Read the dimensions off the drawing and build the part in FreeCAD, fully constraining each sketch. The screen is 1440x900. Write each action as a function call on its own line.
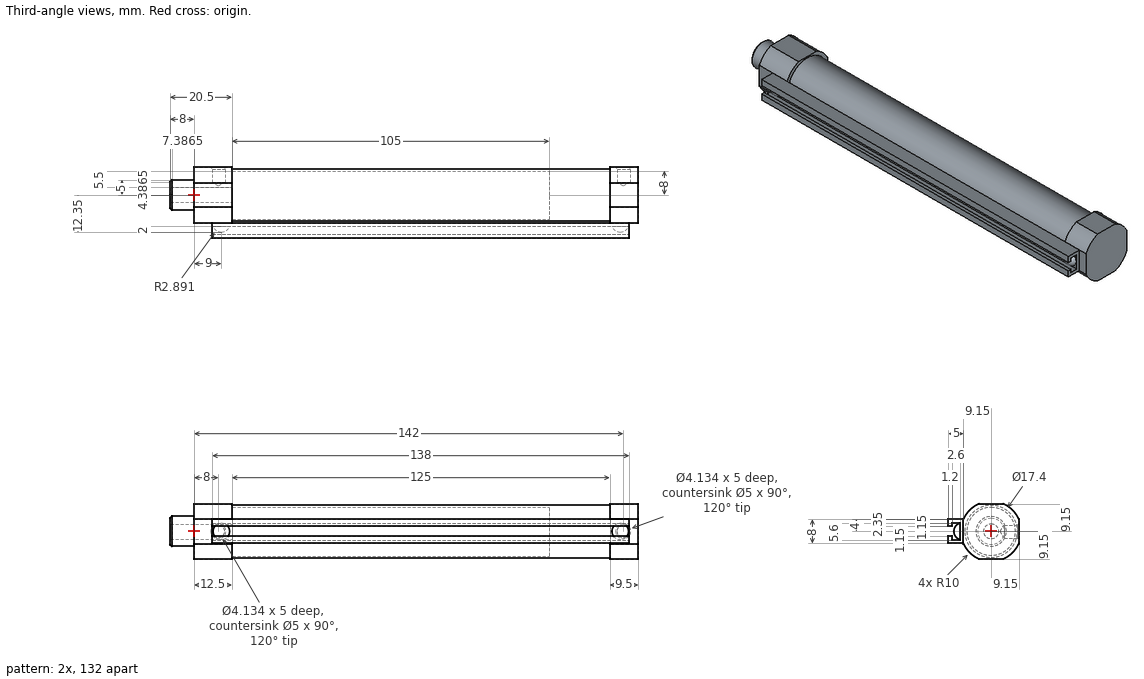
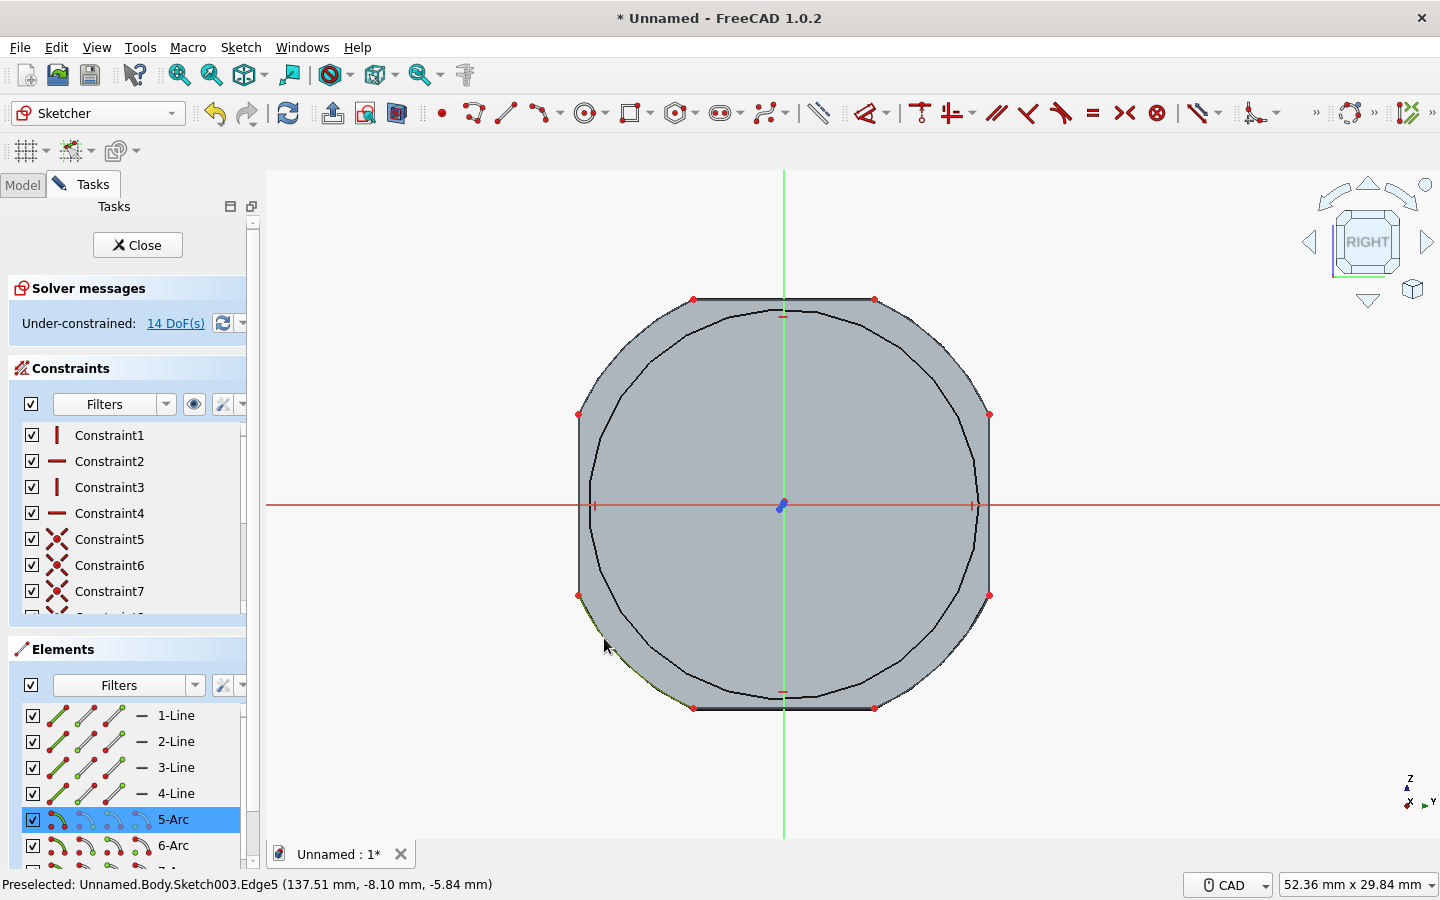
click(964, 372)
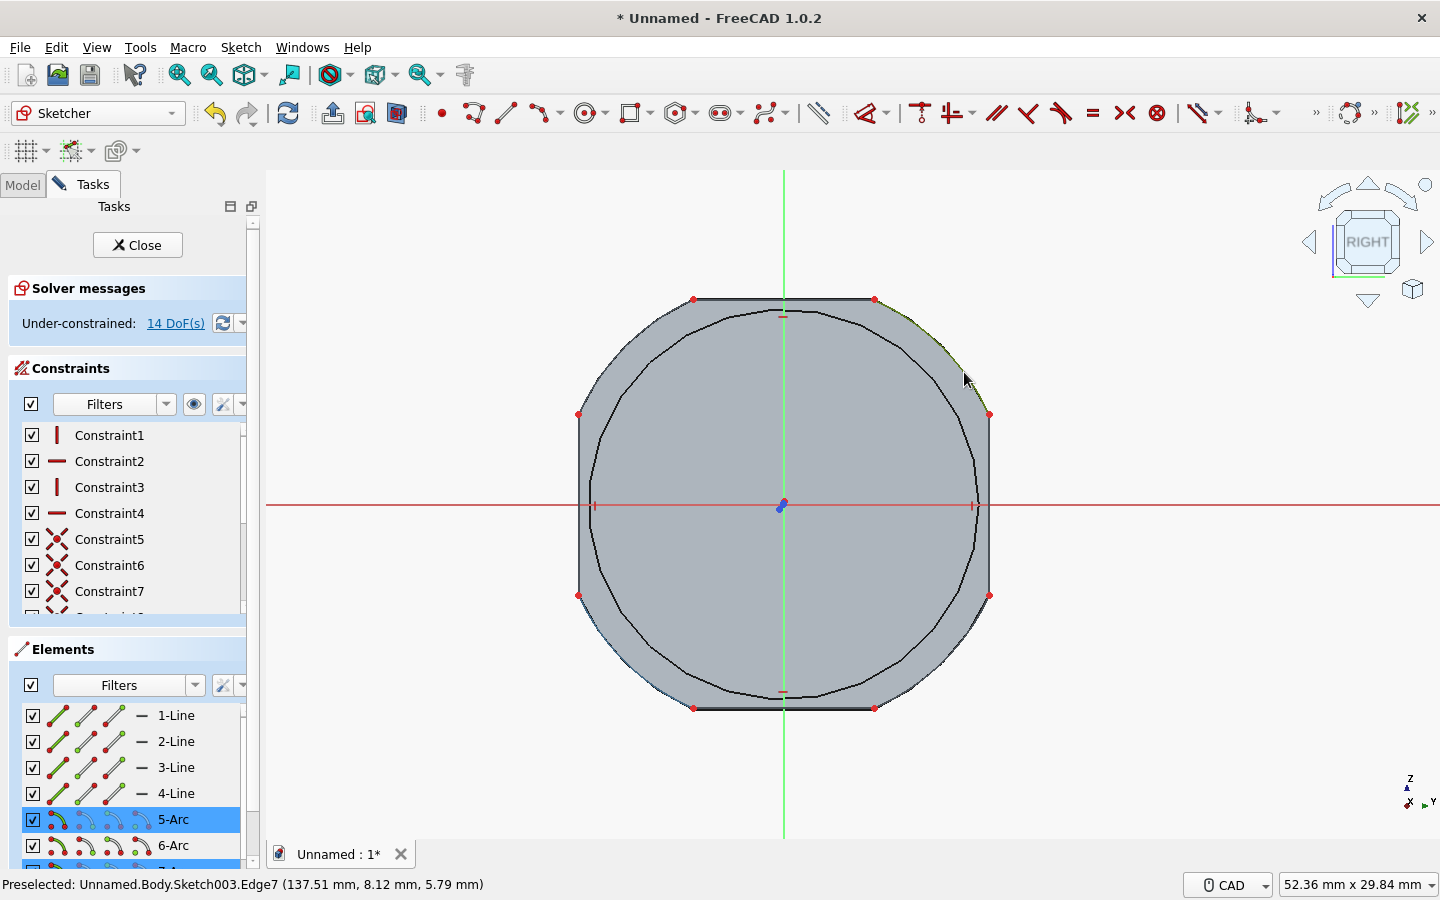
click(920, 114)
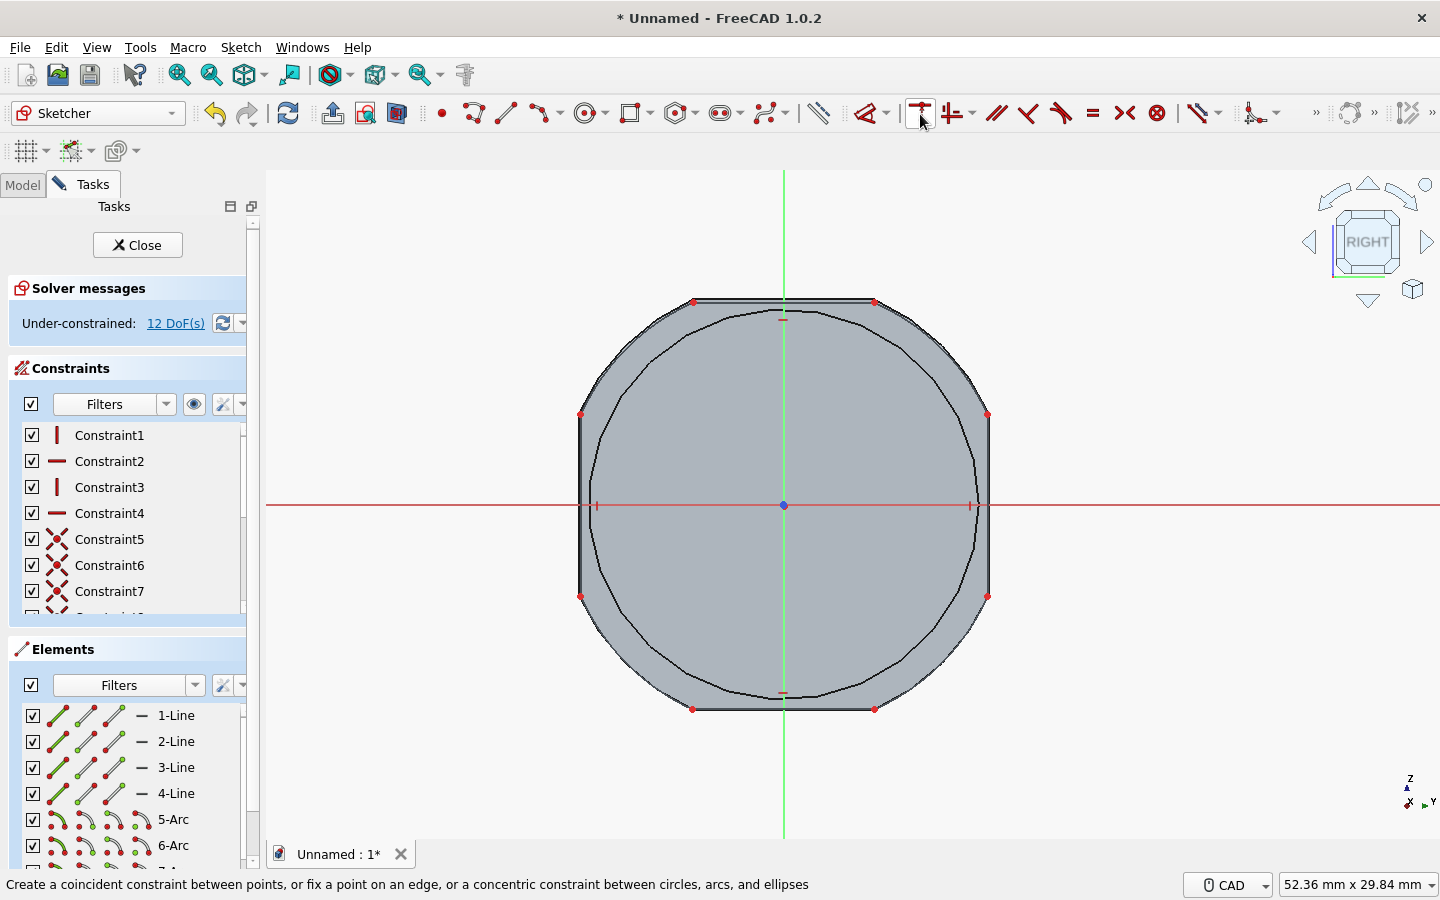
click(605, 638)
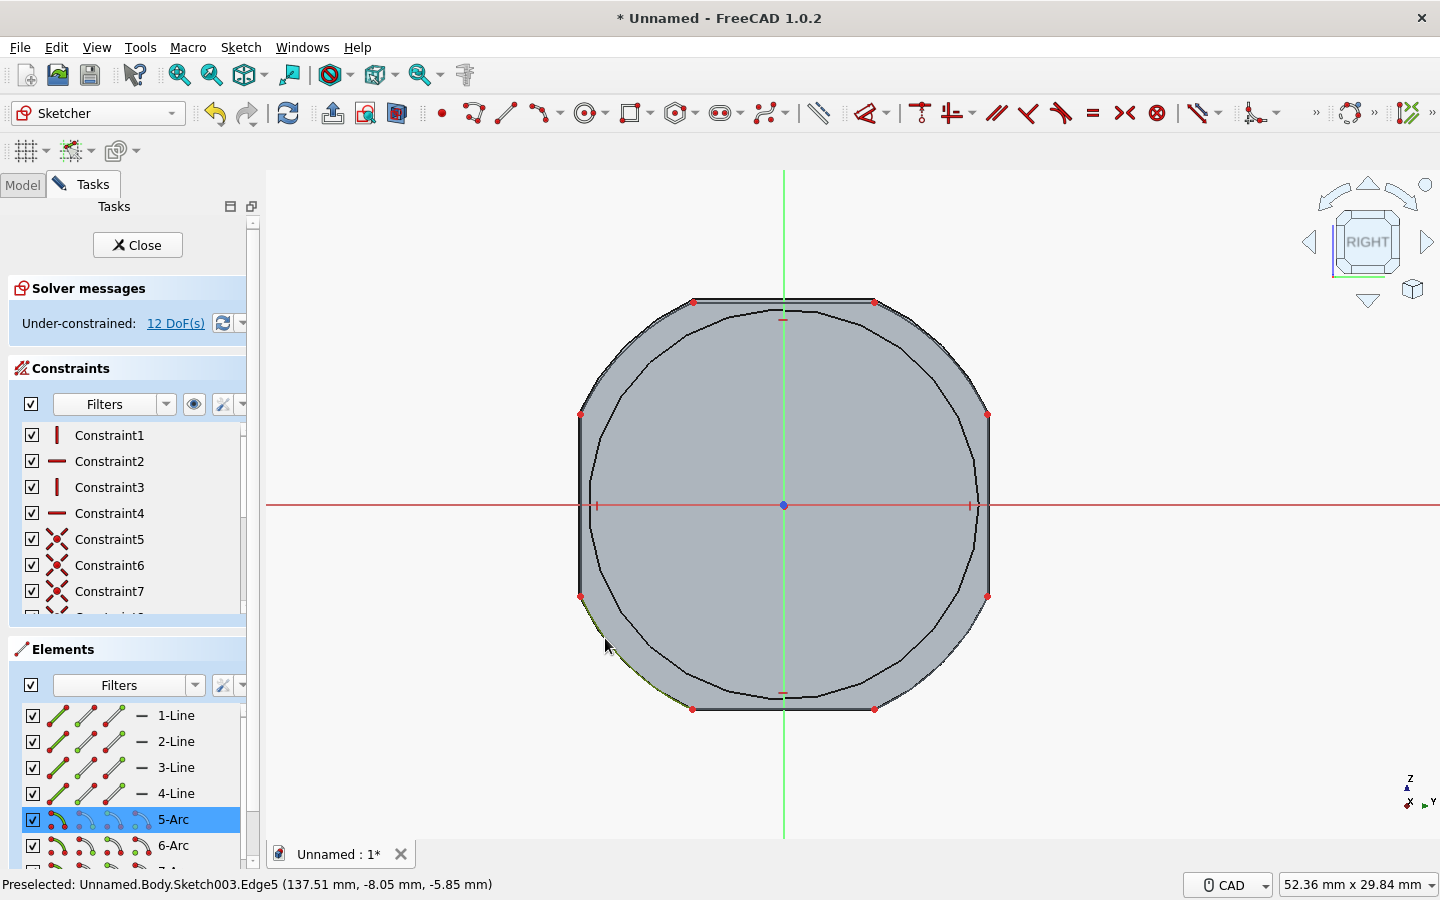
click(651, 327)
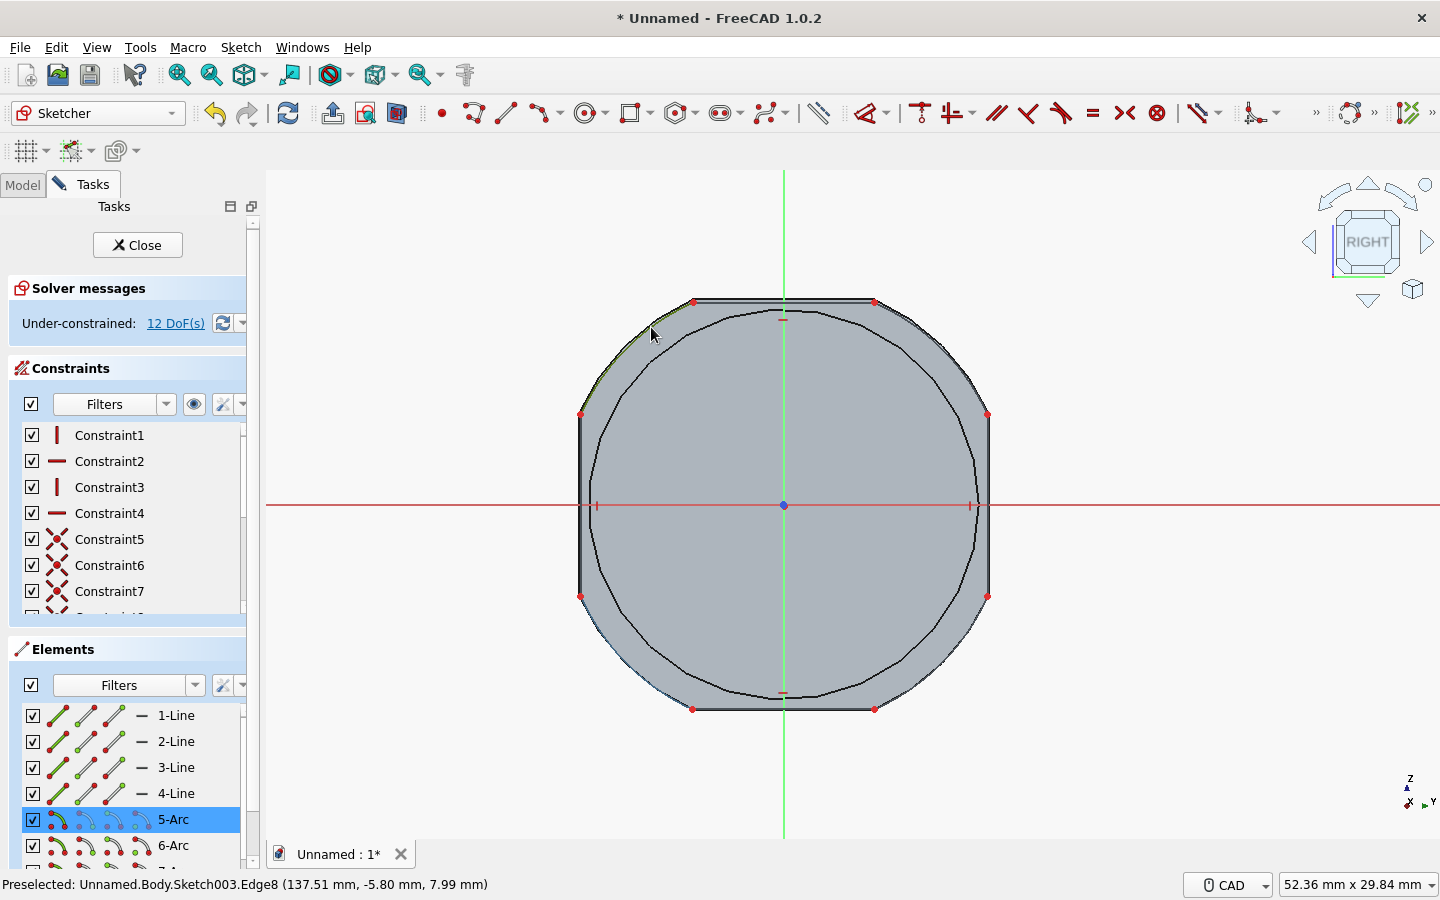
click(920, 114)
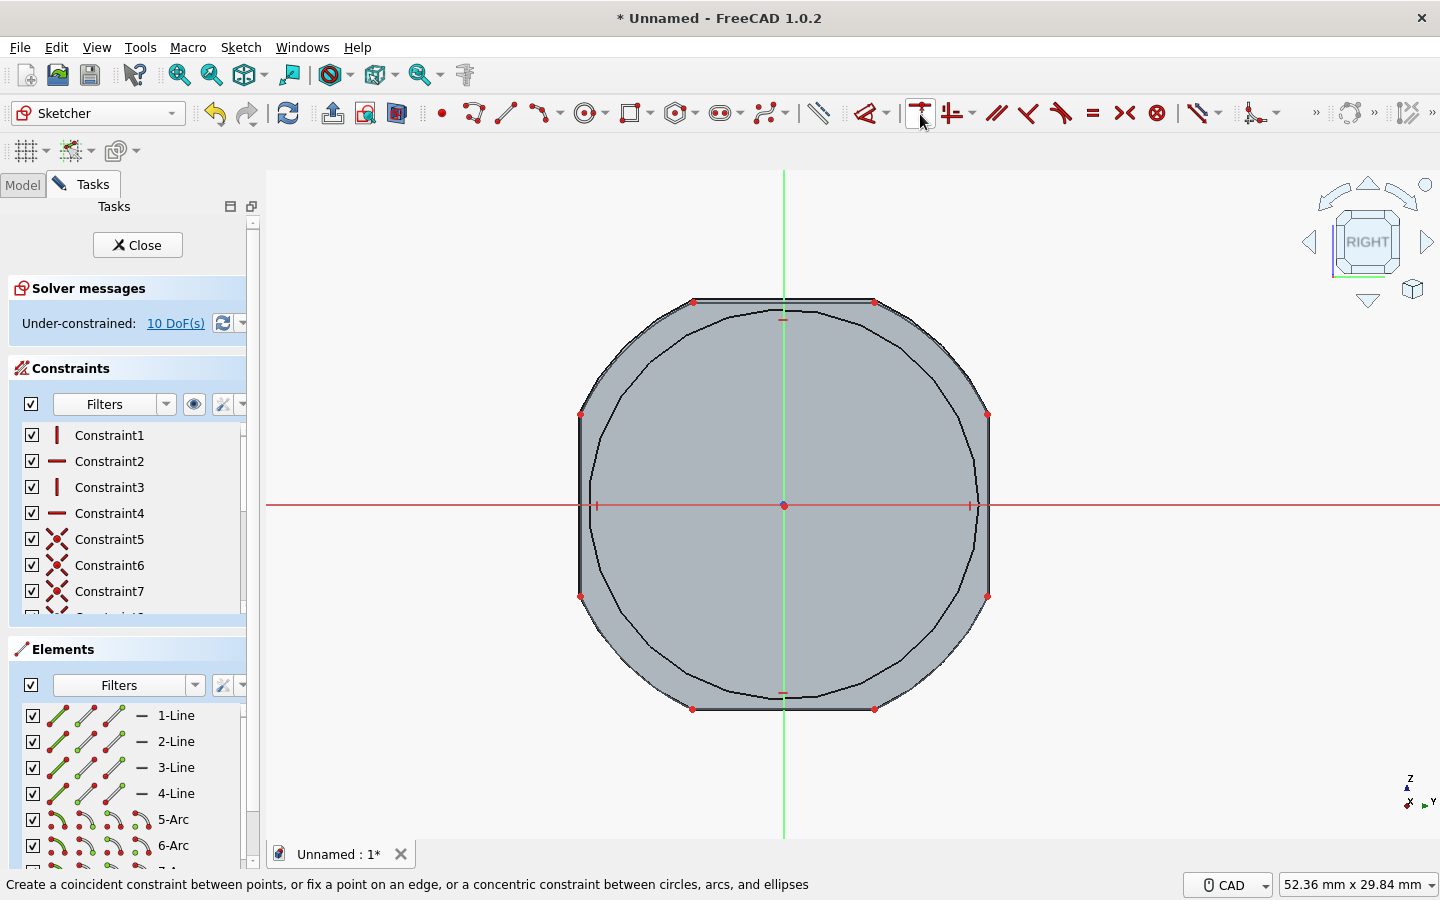
drag(774, 494, 795, 517)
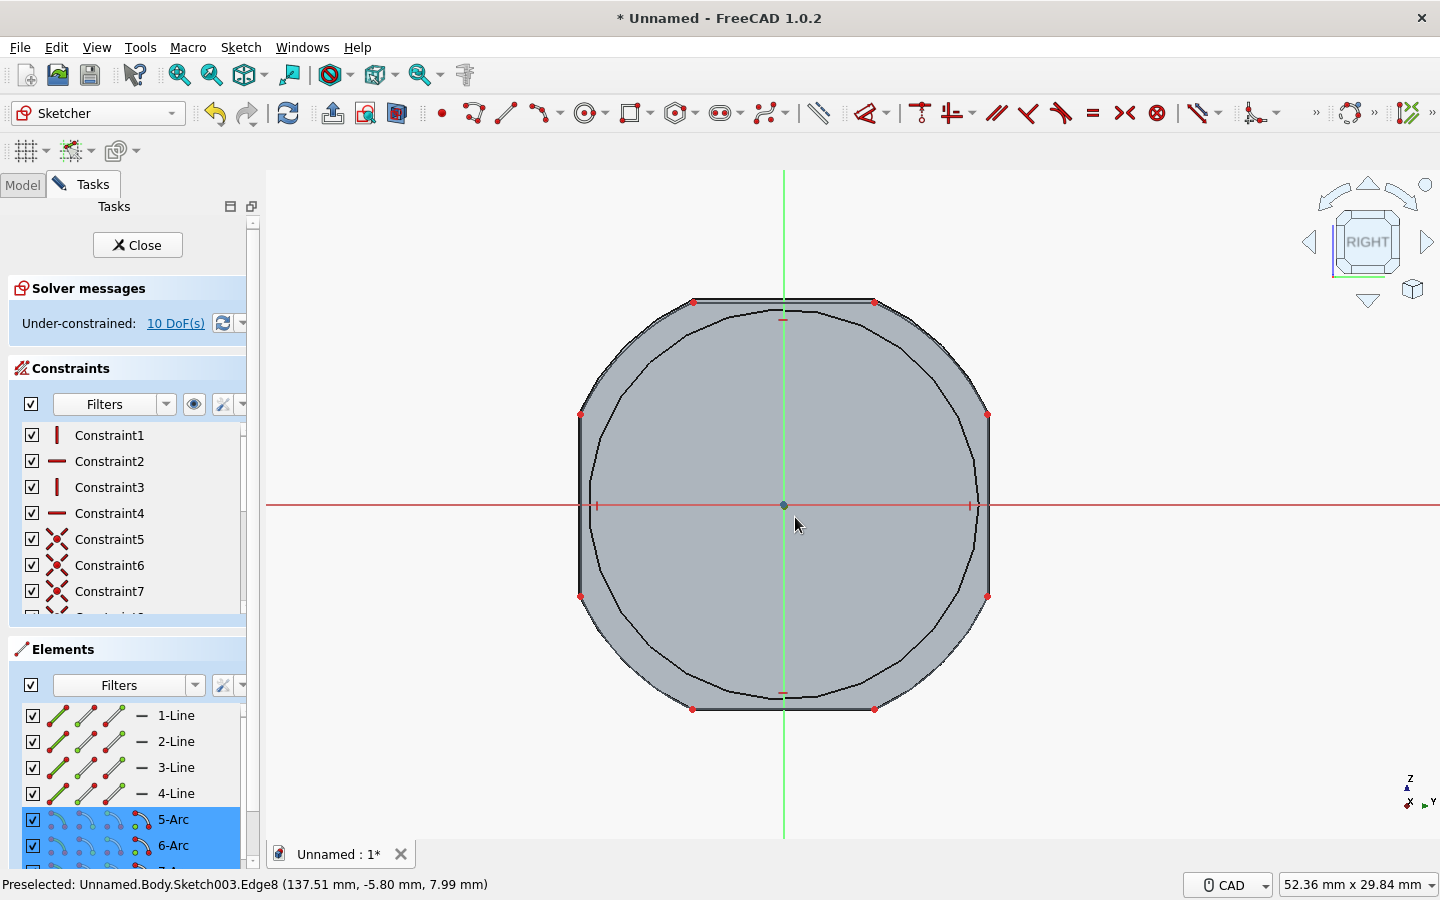
click(920, 114)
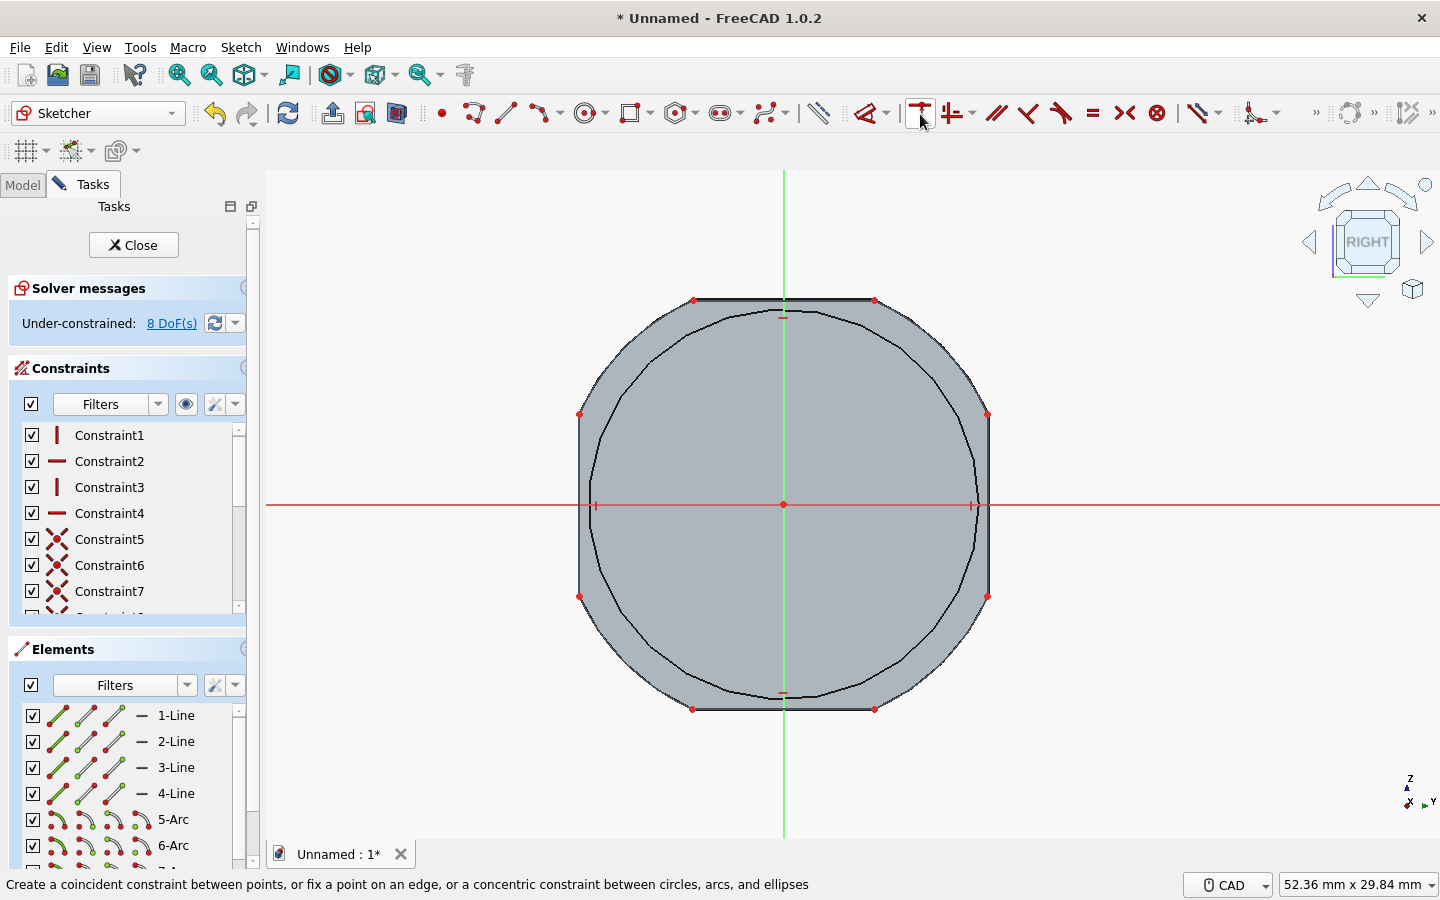
click(604, 638)